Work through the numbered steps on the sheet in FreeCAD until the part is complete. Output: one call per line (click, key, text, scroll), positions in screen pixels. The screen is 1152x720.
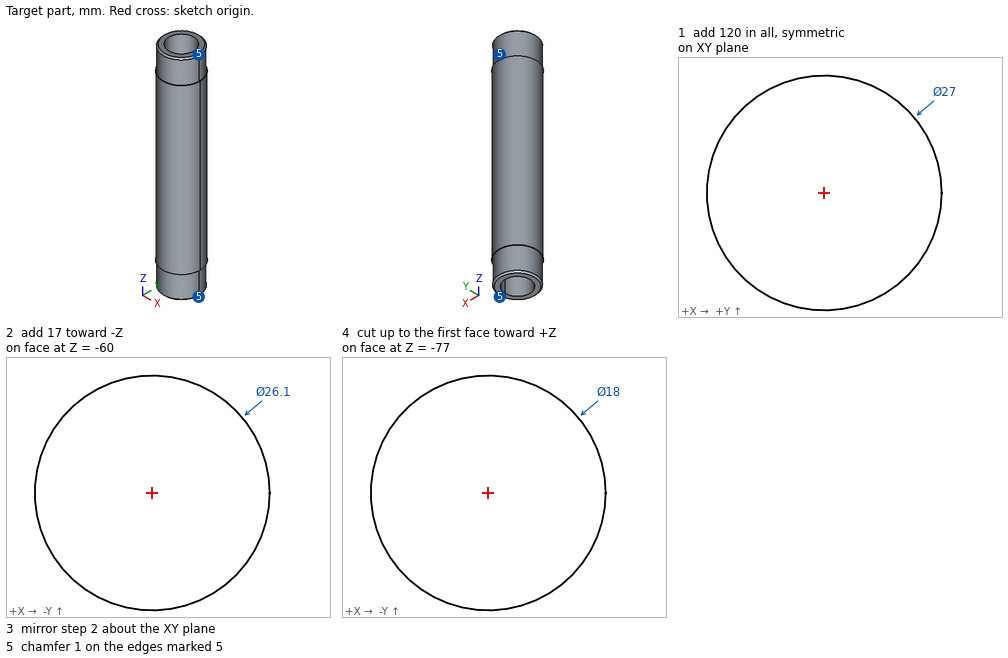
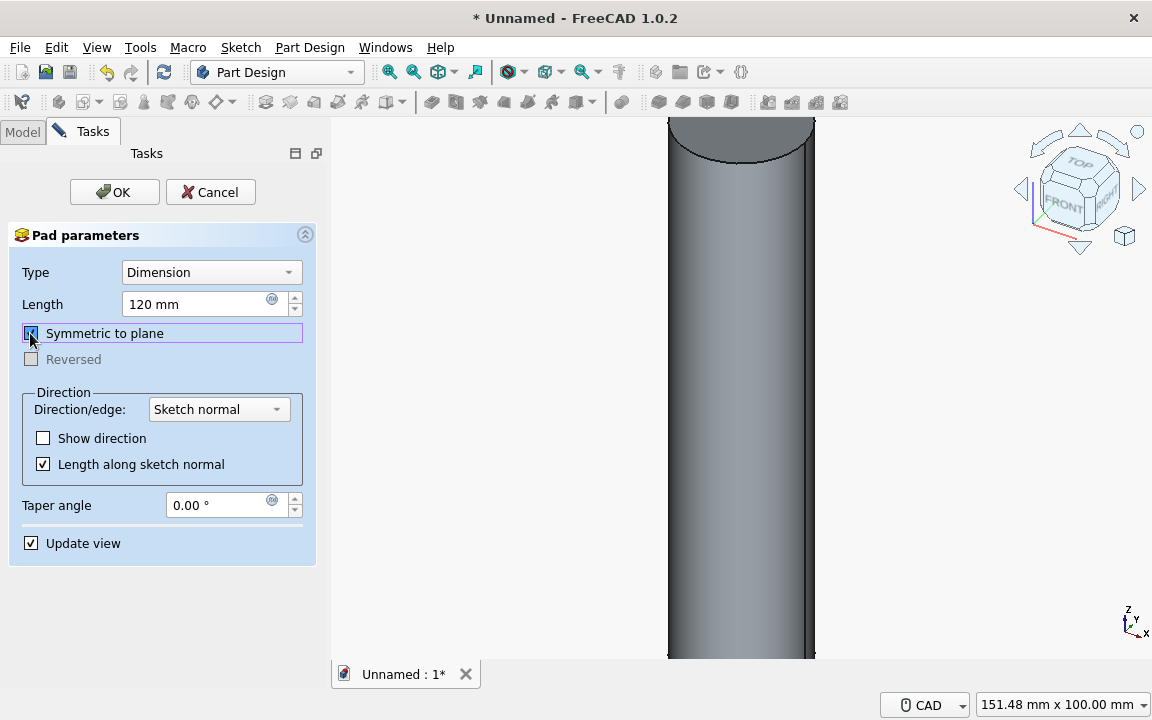
click(115, 192)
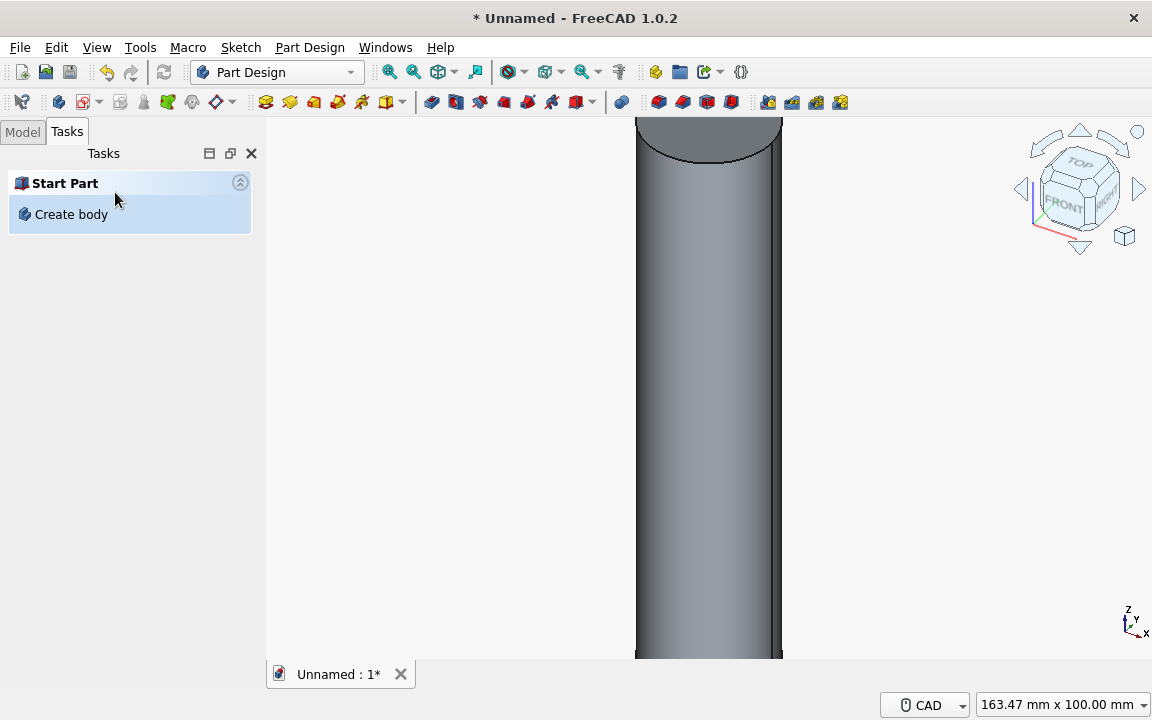
key(v)
key(f)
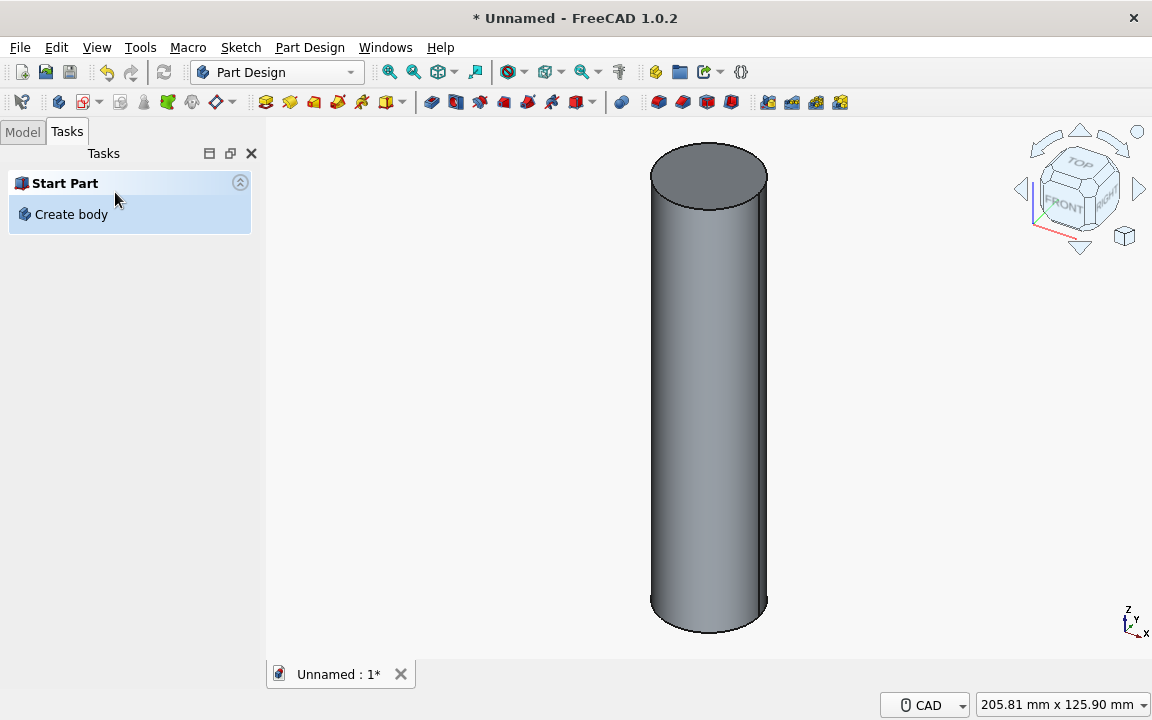
key(5)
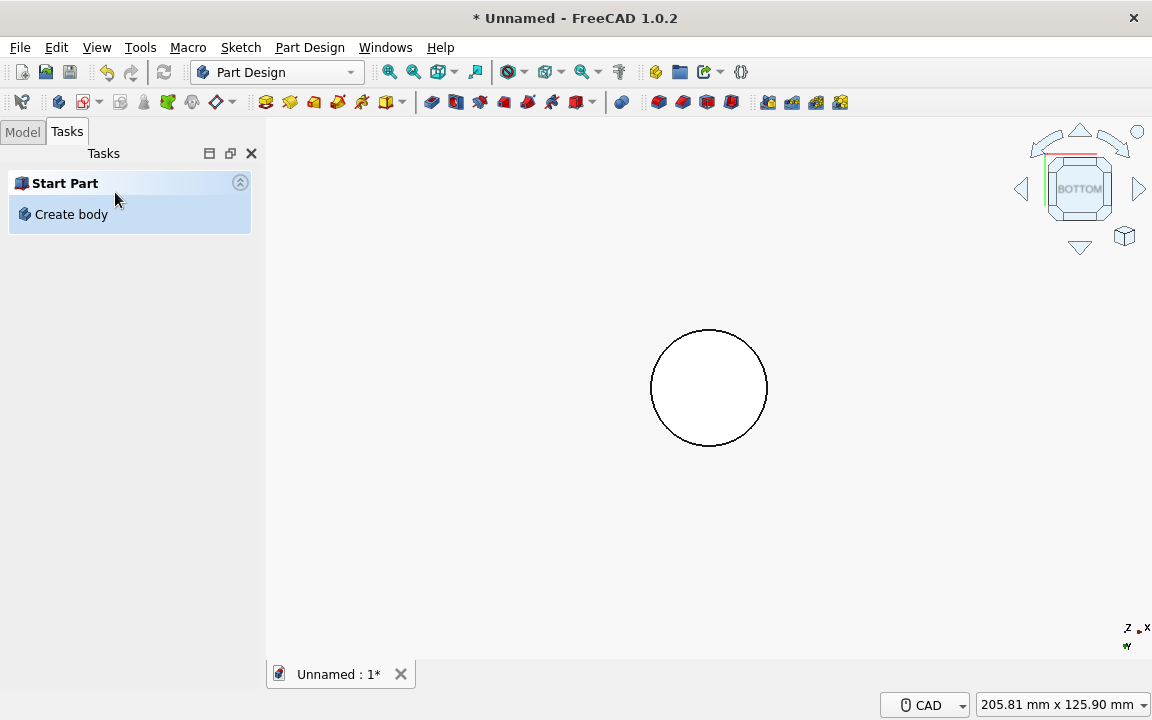
key(v)
key(f)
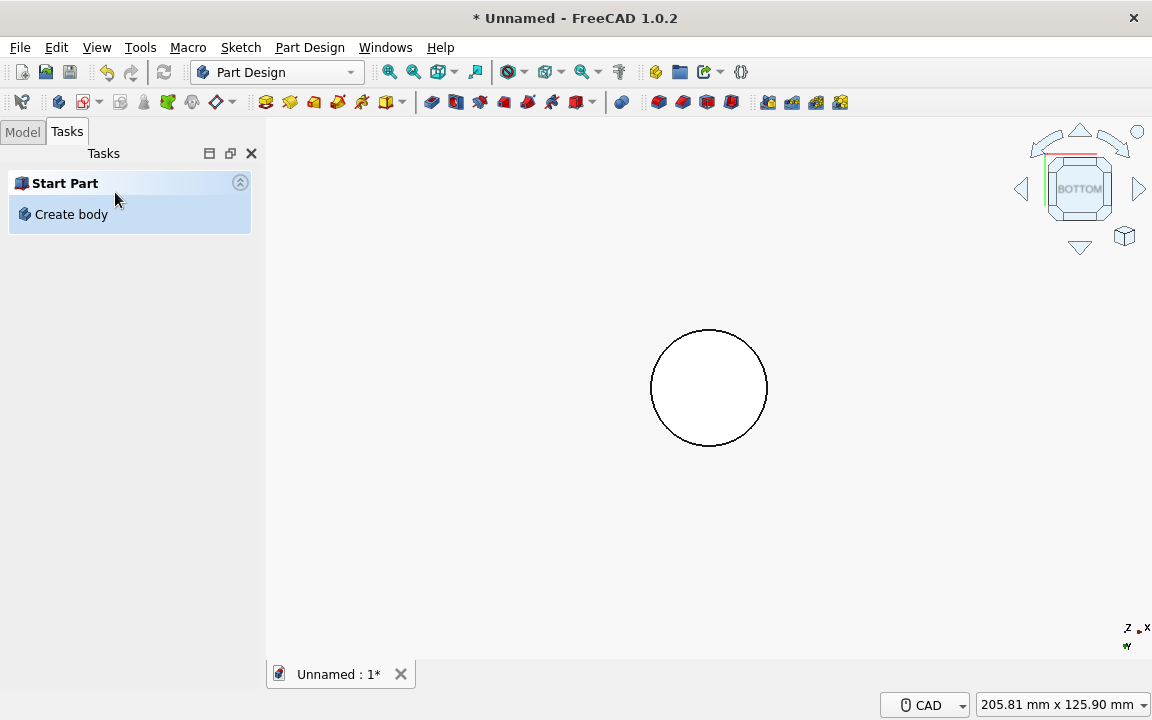
click(709, 387)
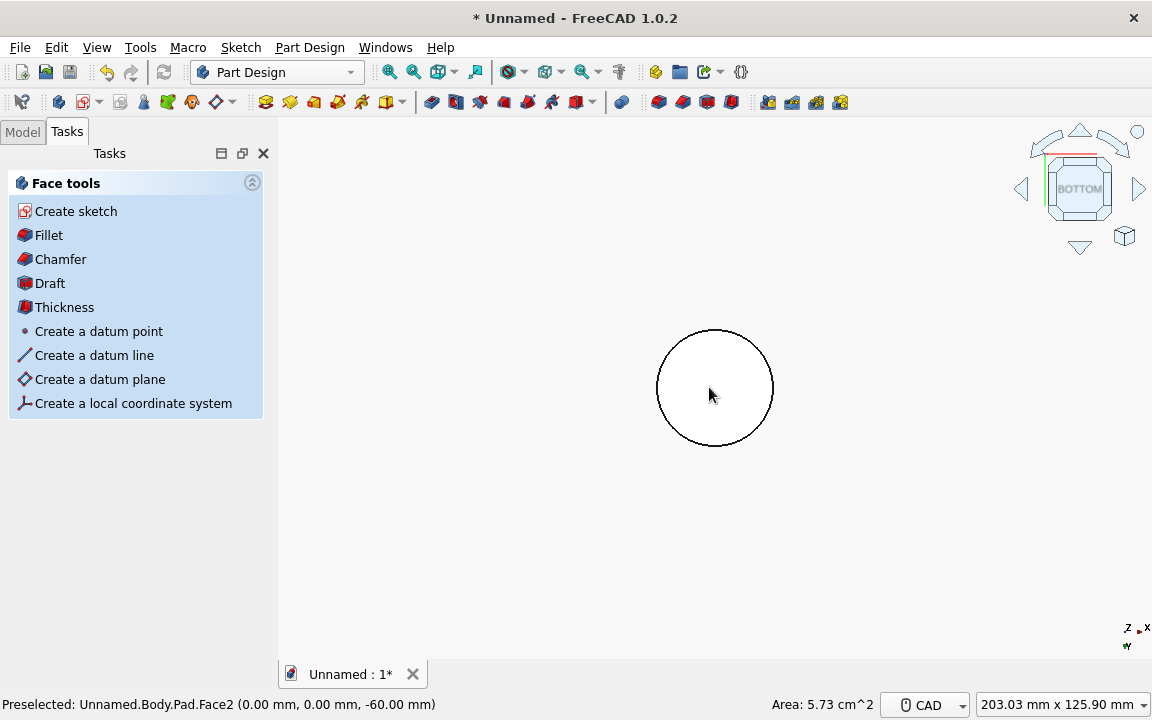
click(84, 102)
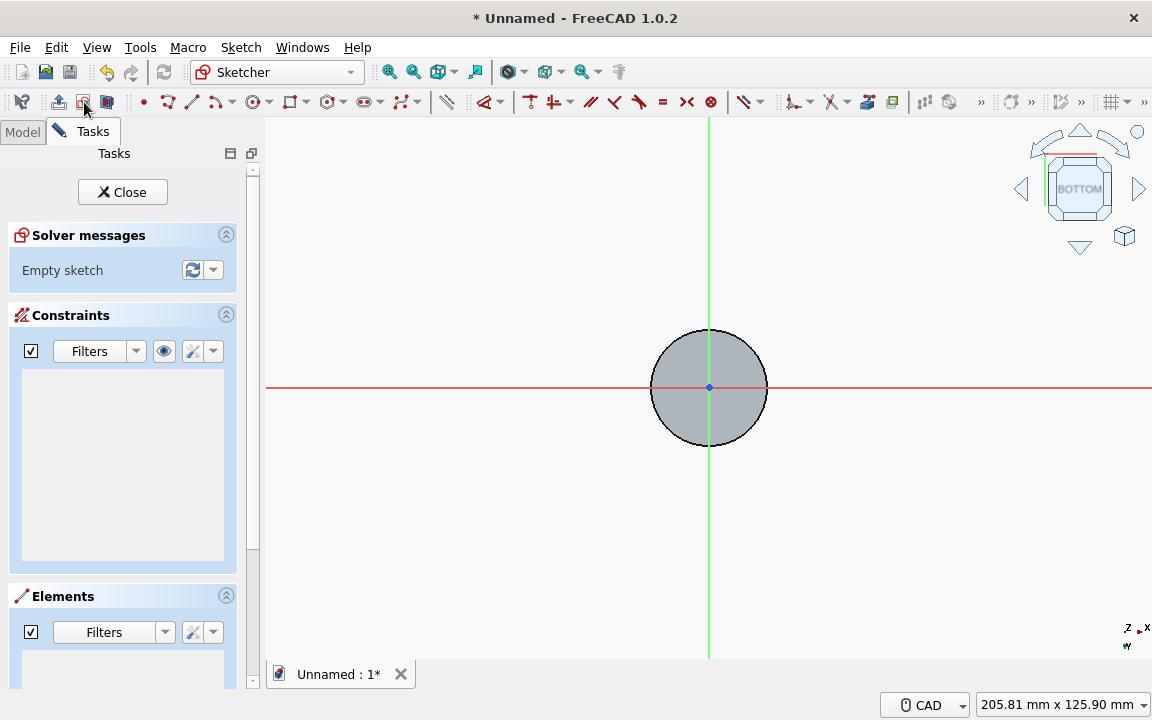
scroll(739, 388, up, 6)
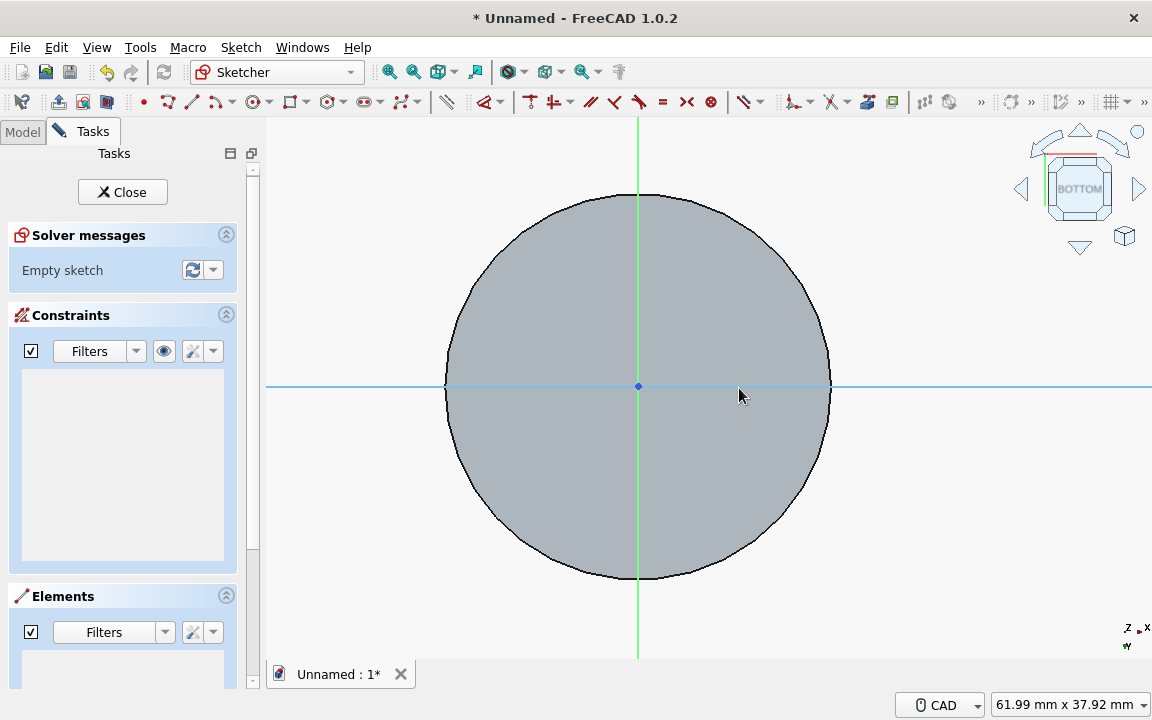
click(254, 102)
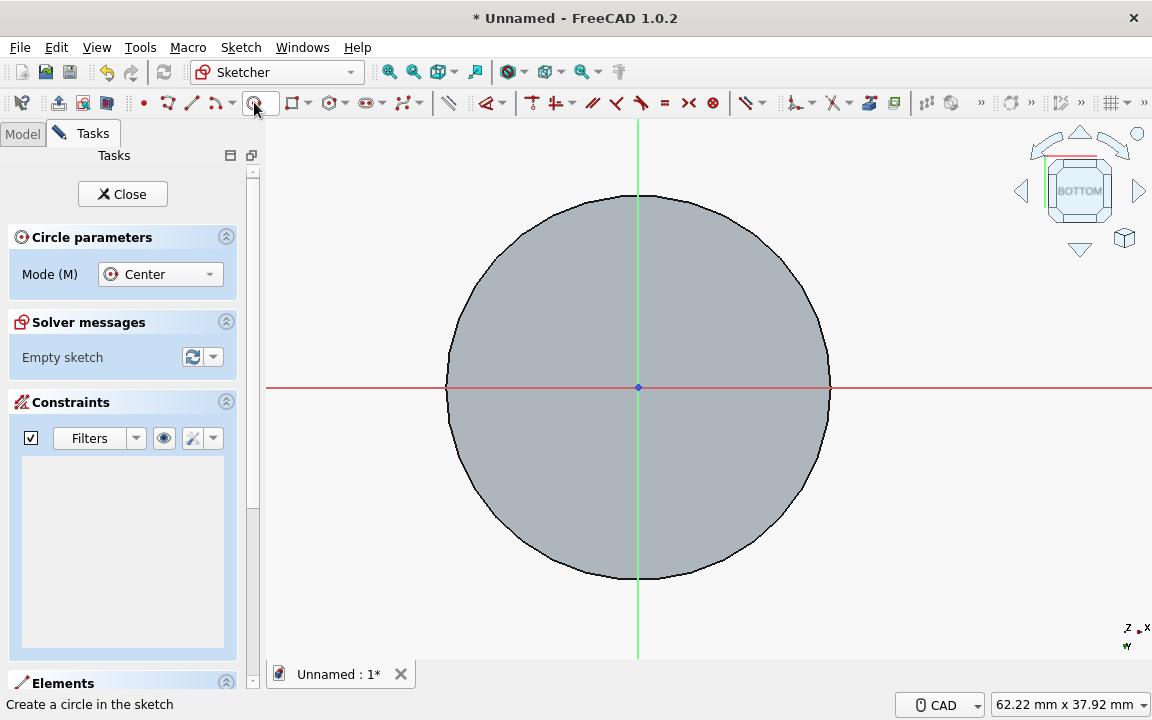
click(638, 388)
move(770, 256)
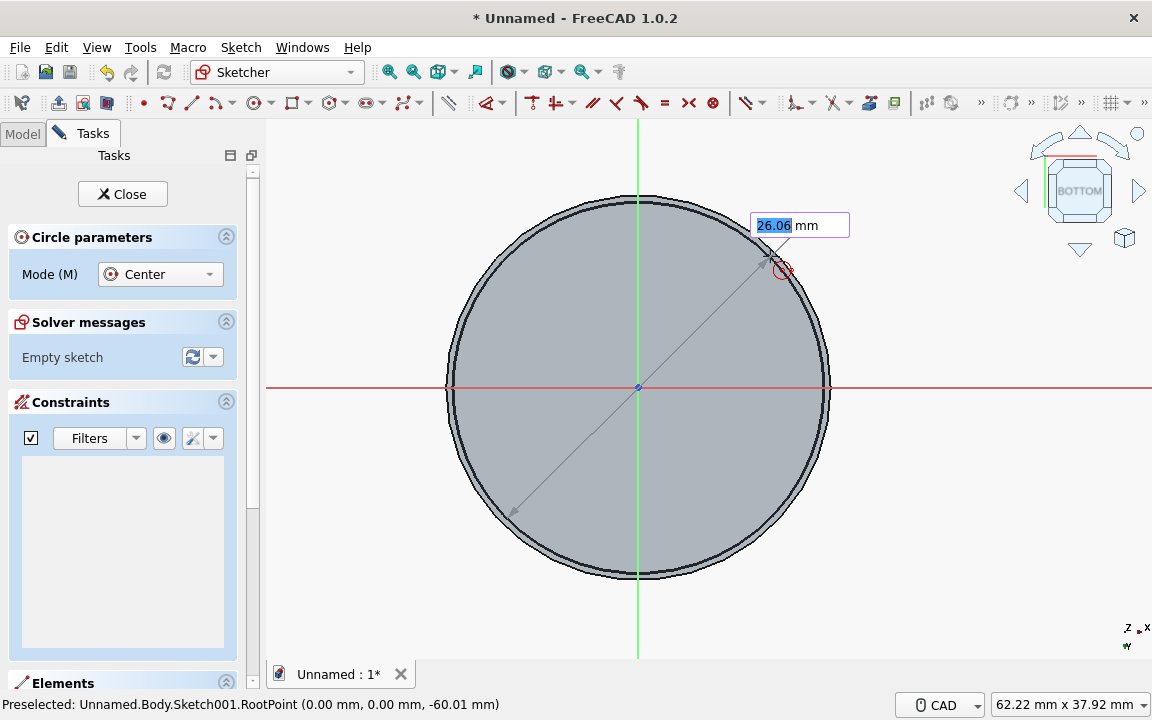
text(26.1)
key(Return)
key(Escape)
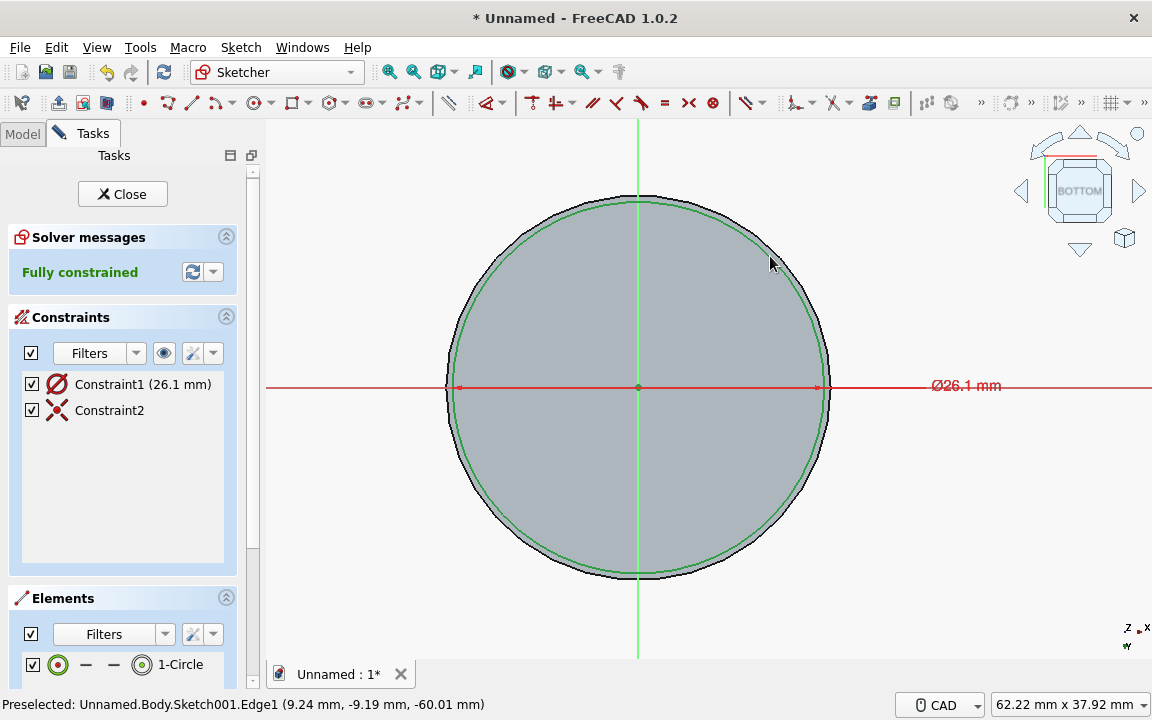
click(123, 194)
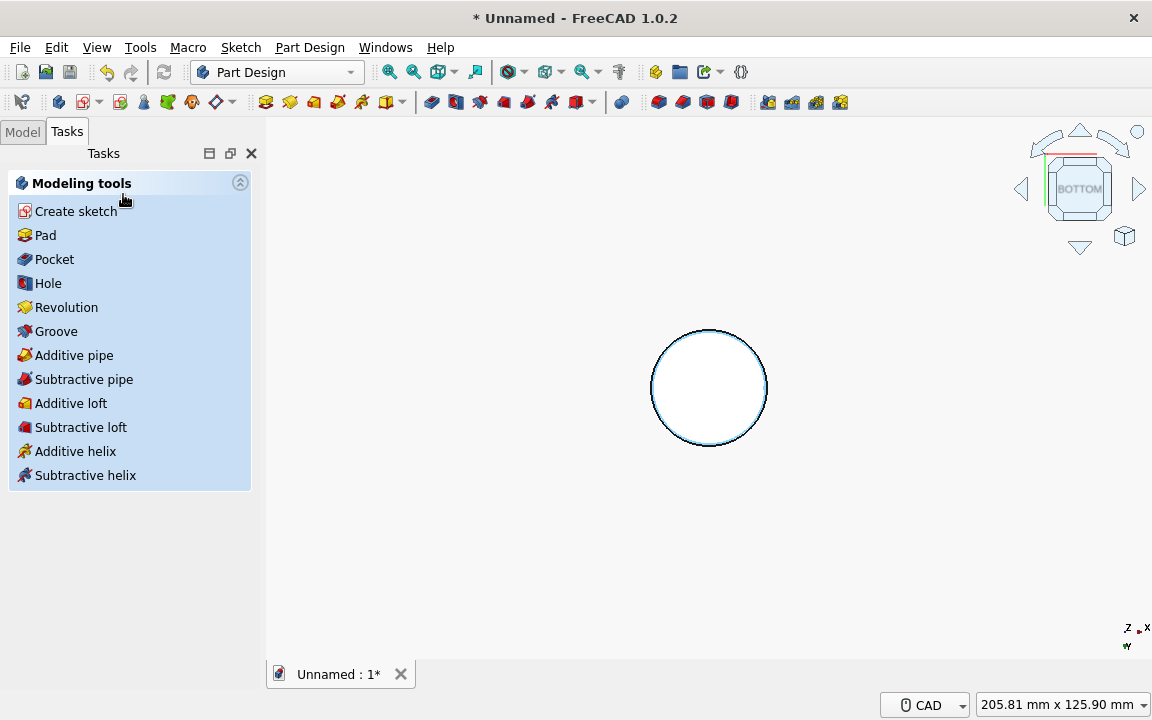
click(266, 102)